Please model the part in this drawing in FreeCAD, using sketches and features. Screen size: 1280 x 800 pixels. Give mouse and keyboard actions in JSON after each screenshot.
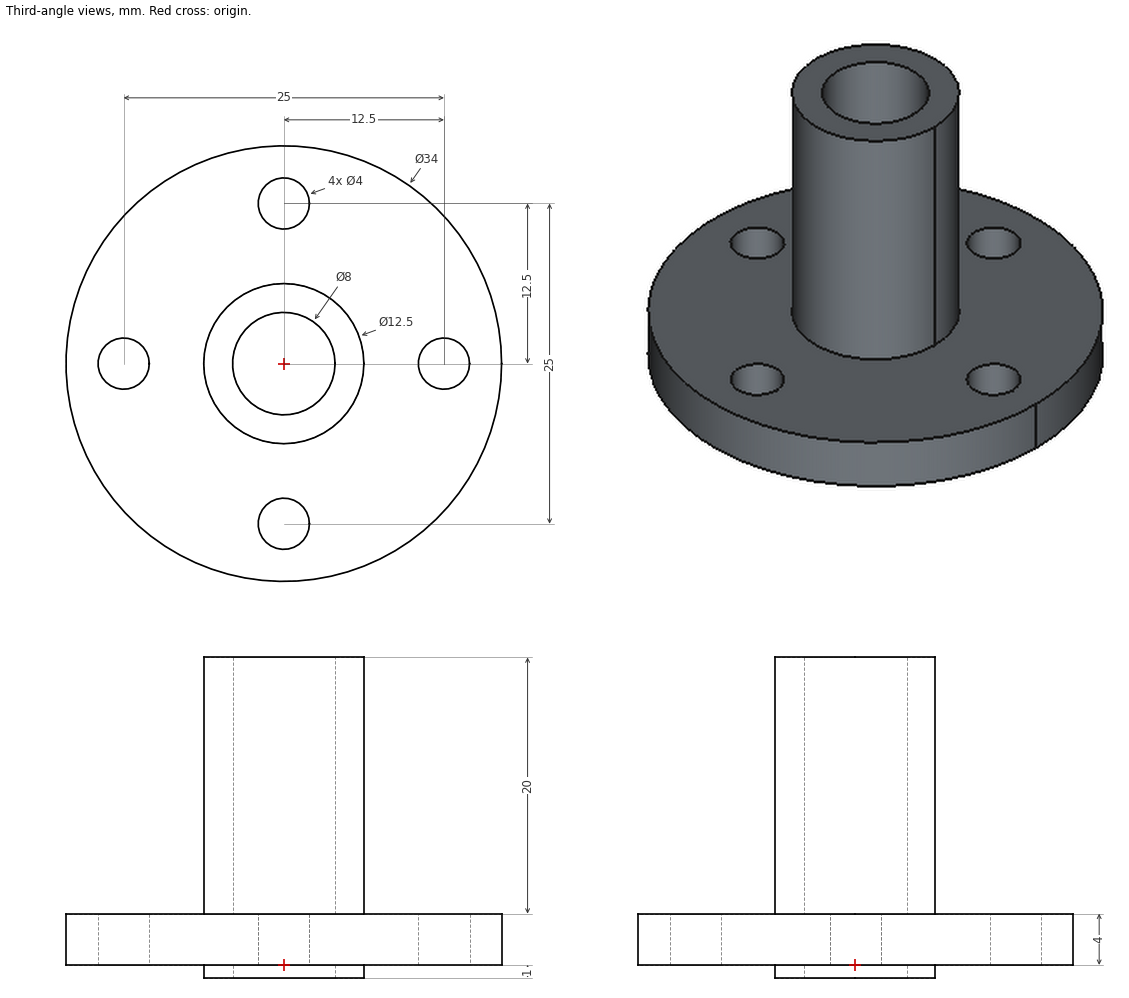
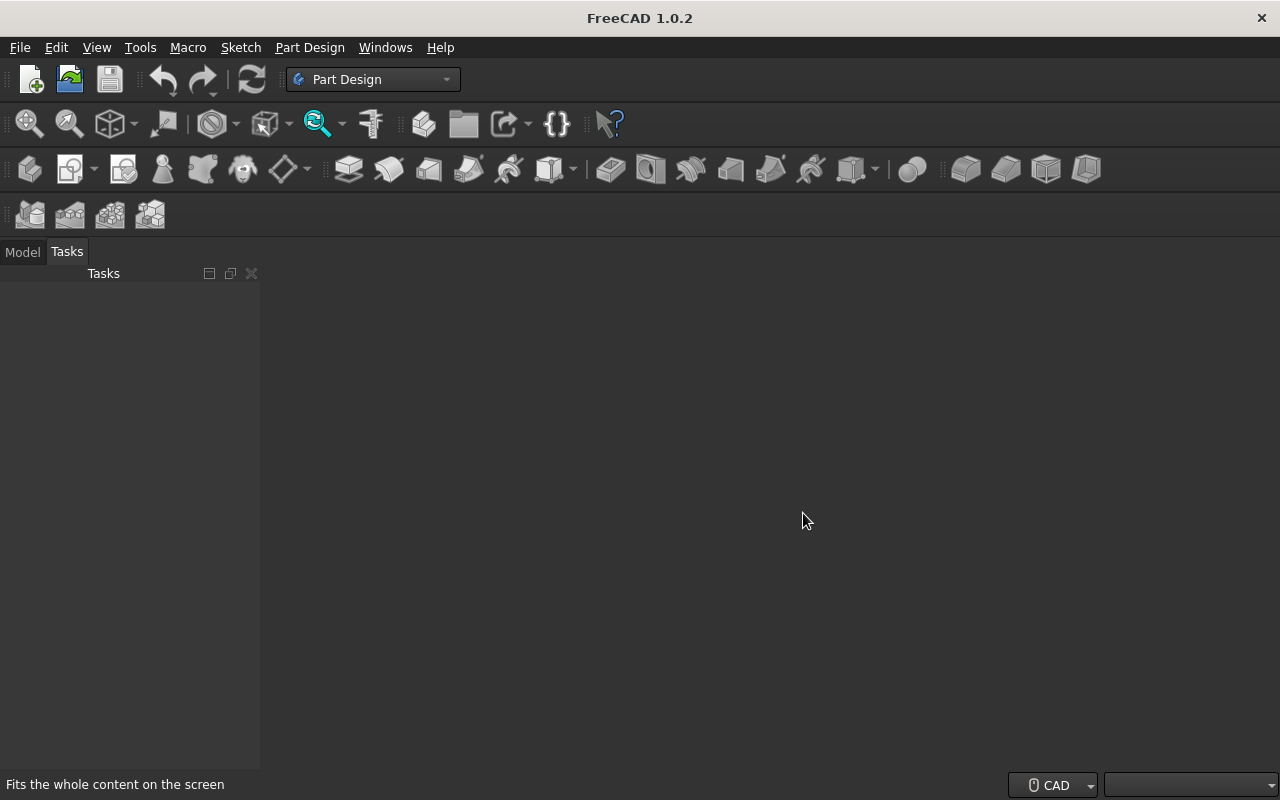
{"action": "left_click", "coordinate": [30, 80]}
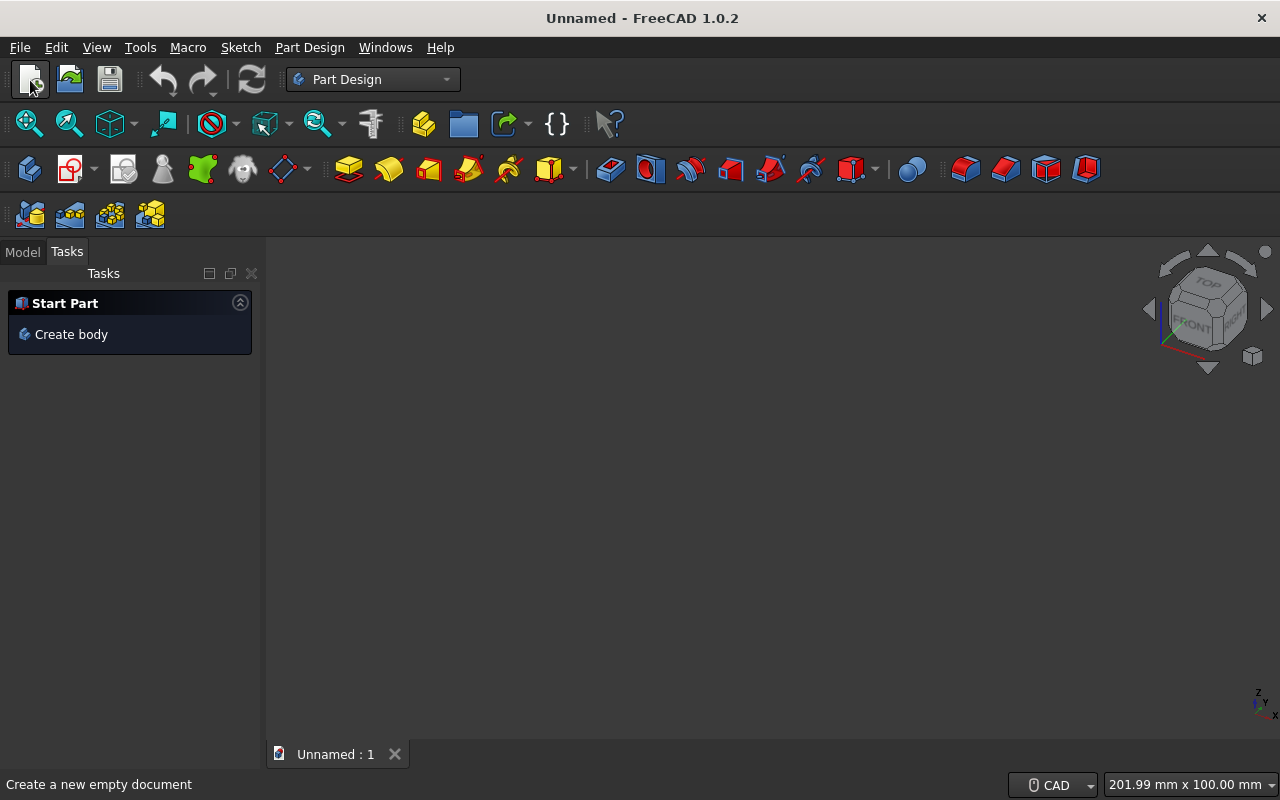
{"action": "left_click", "coordinate": [70, 170]}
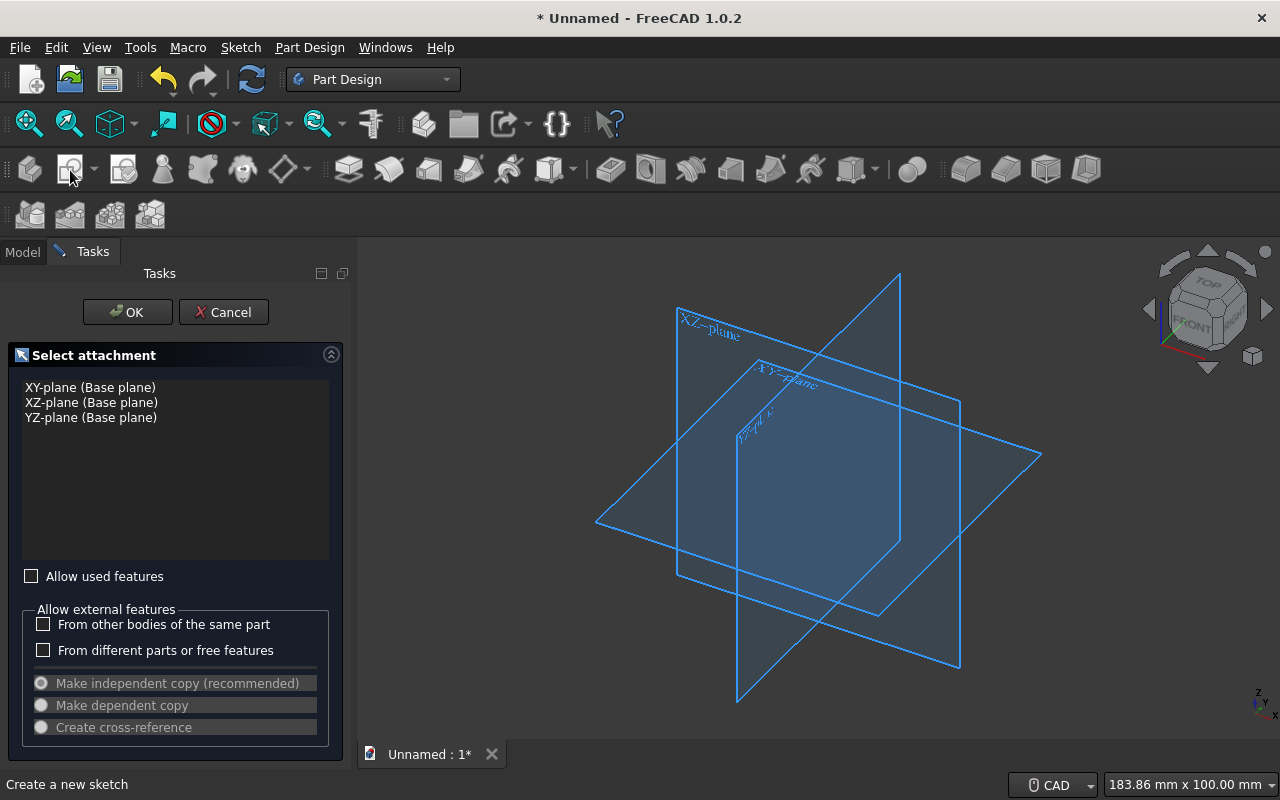
{"action": "left_click", "coordinate": [82, 388]}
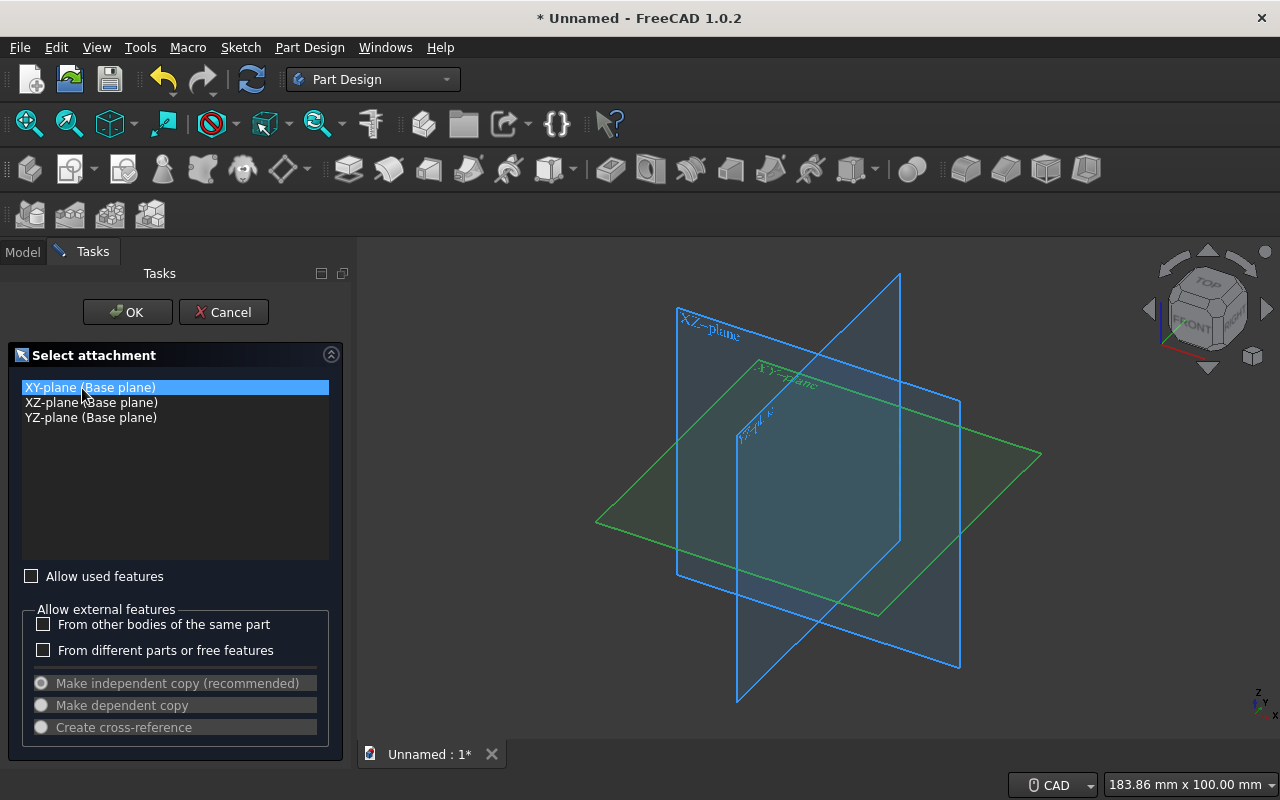
{"action": "left_click", "coordinate": [128, 312]}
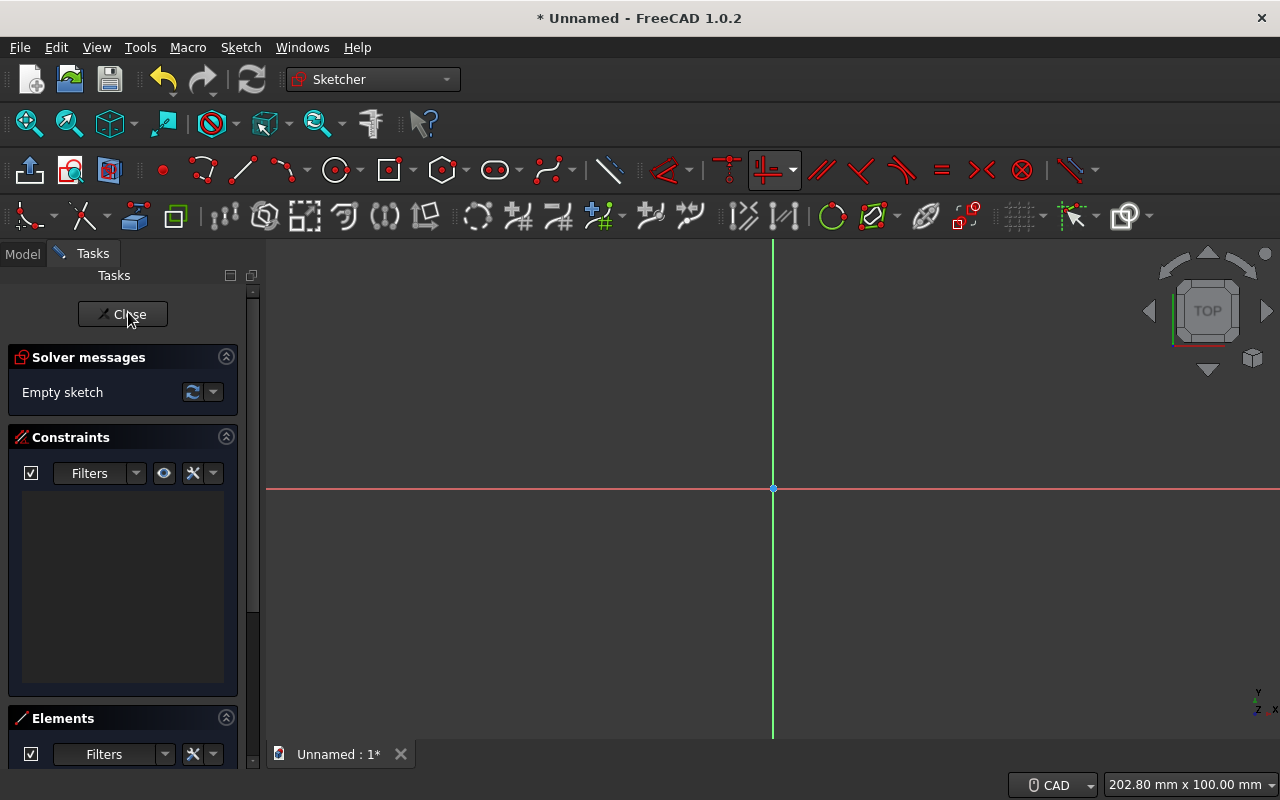
{"action": "scroll", "coordinate": [856, 489], "scroll_direction": "up", "scroll_amount": 3}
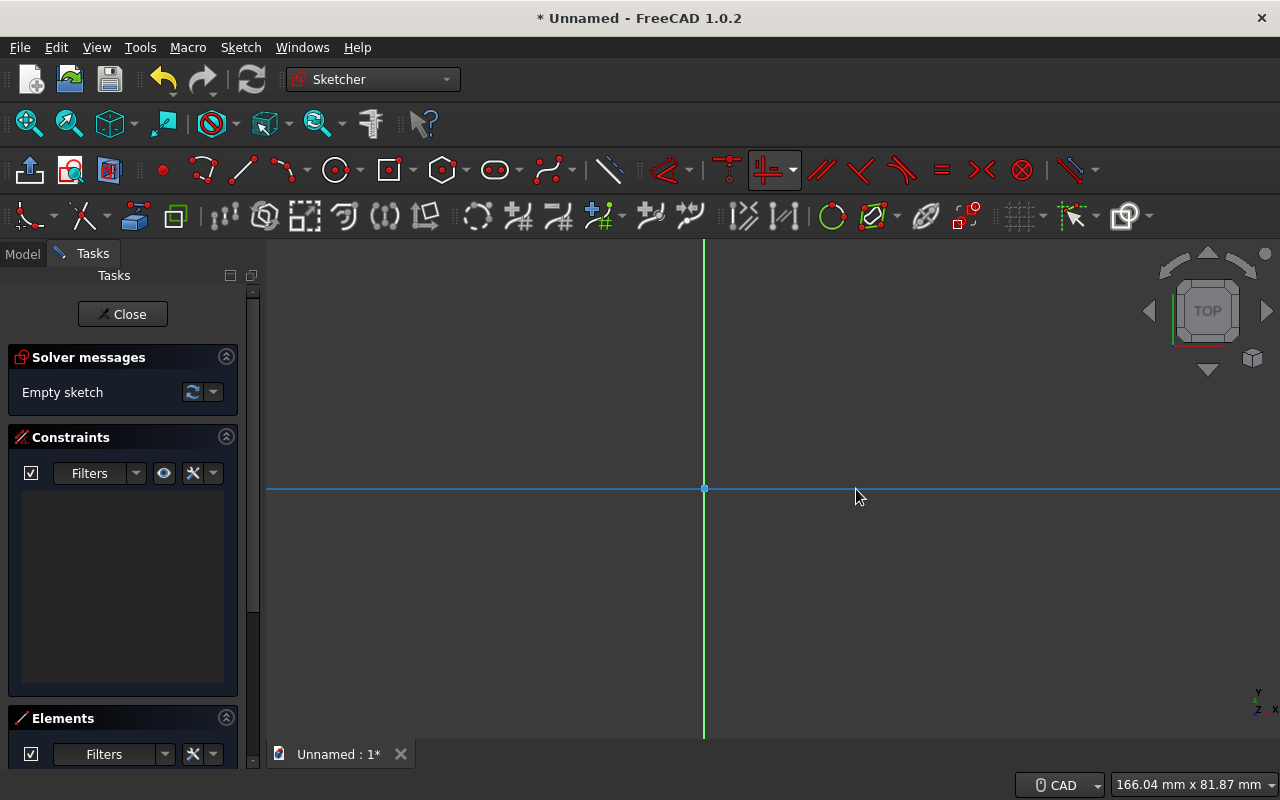
{"action": "left_click", "coordinate": [336, 170]}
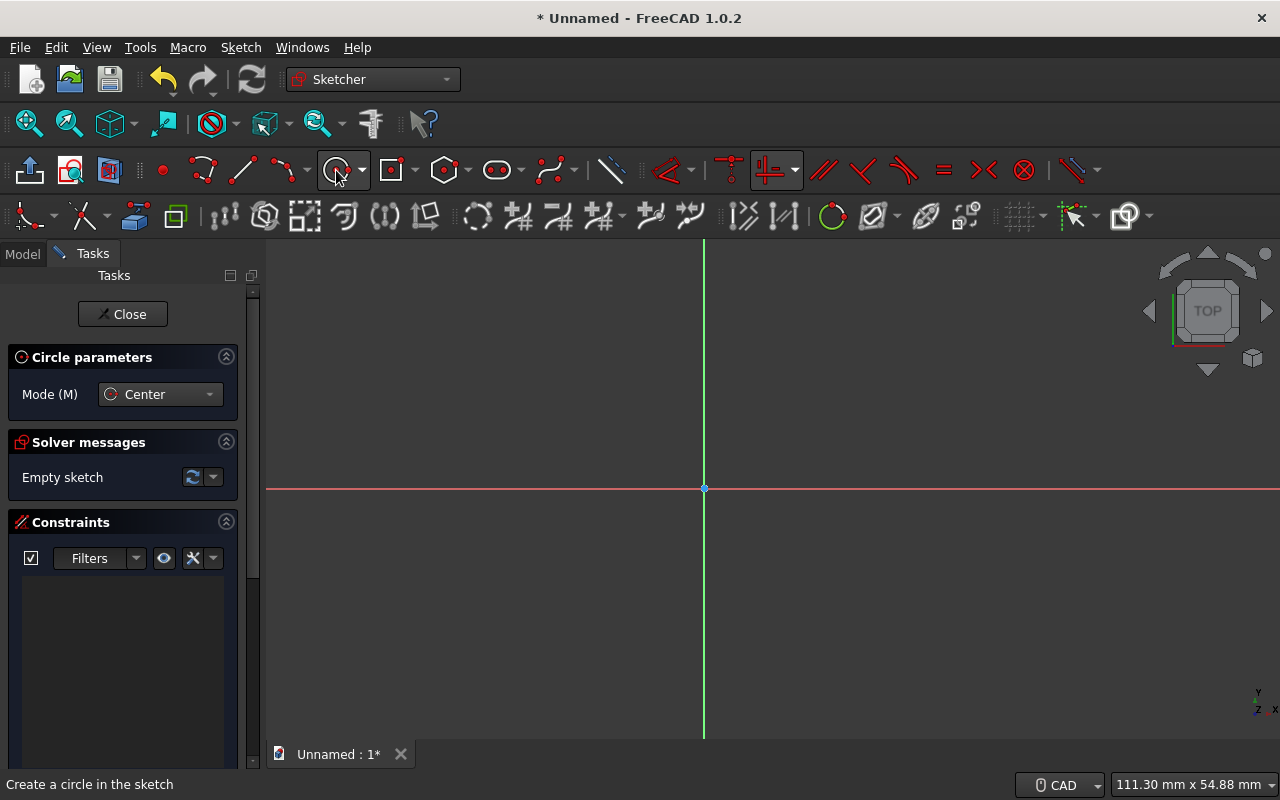
{"action": "left_click", "coordinate": [704, 489]}
{"action": "mouse_move", "coordinate": [814, 379]}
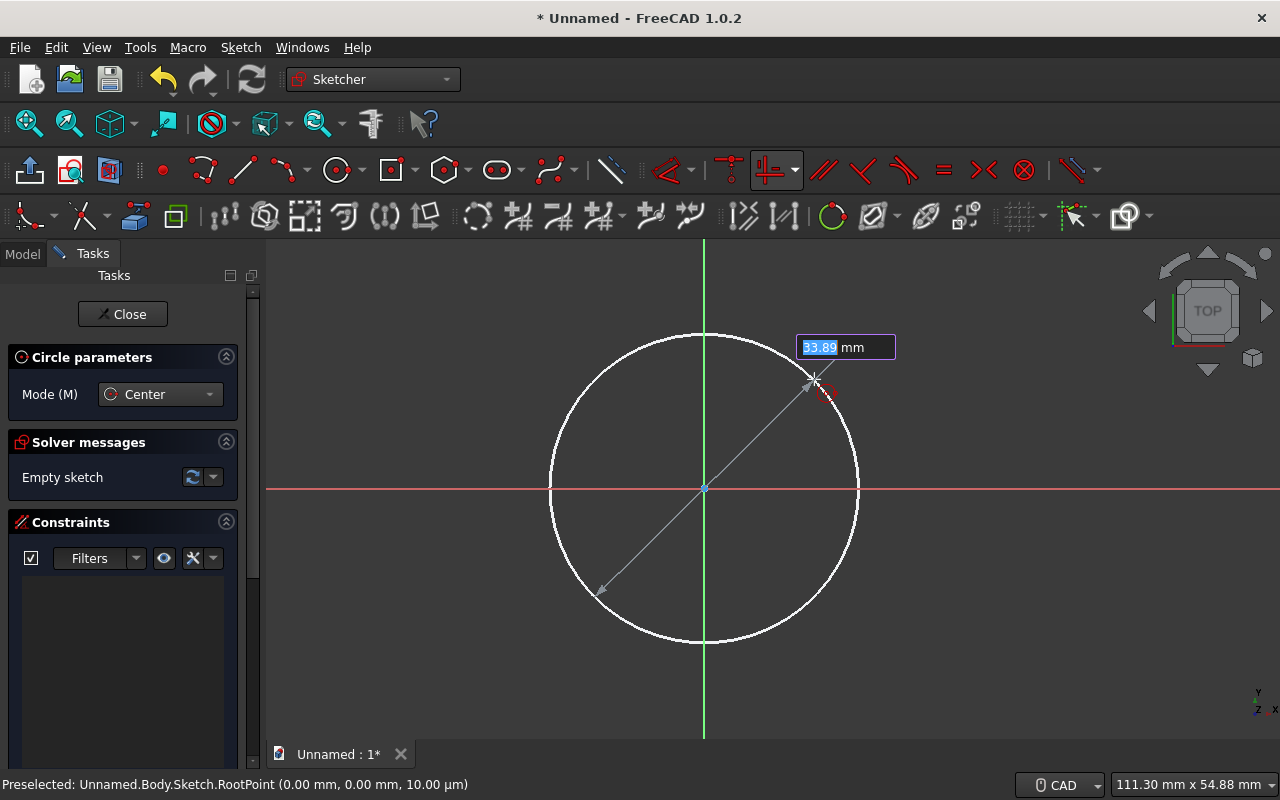
{"action": "type", "text": "34"}
{"action": "key", "text": "Return"}
{"action": "key", "text": "Escape"}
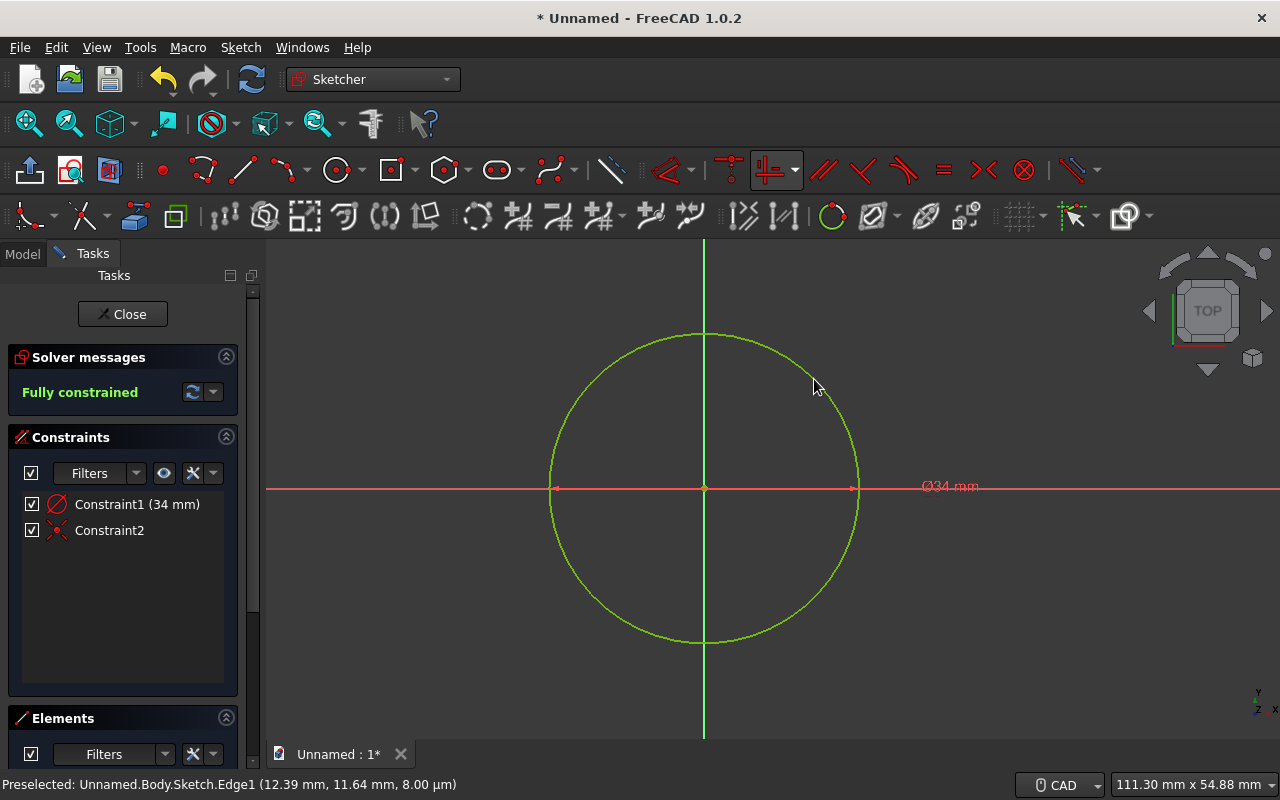
{"action": "left_click", "coordinate": [123, 314]}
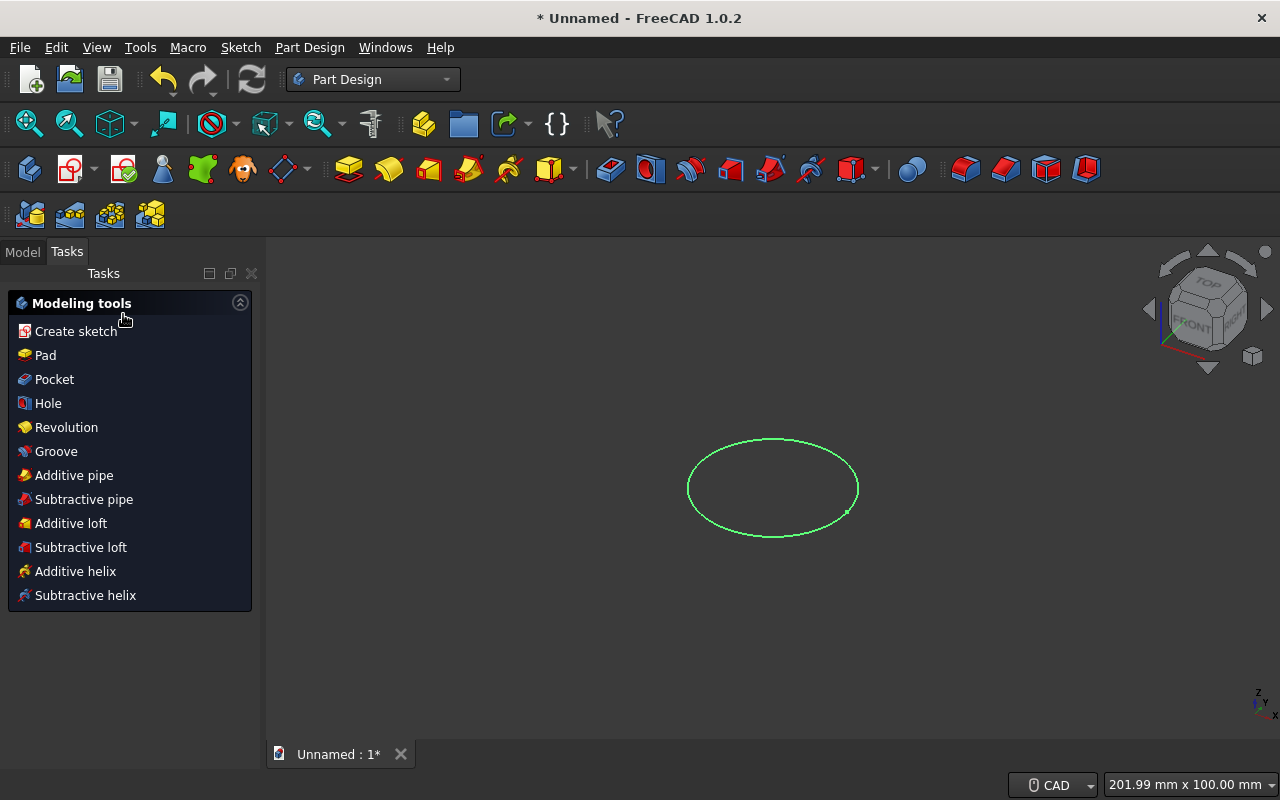
{"action": "left_click", "coordinate": [350, 170]}